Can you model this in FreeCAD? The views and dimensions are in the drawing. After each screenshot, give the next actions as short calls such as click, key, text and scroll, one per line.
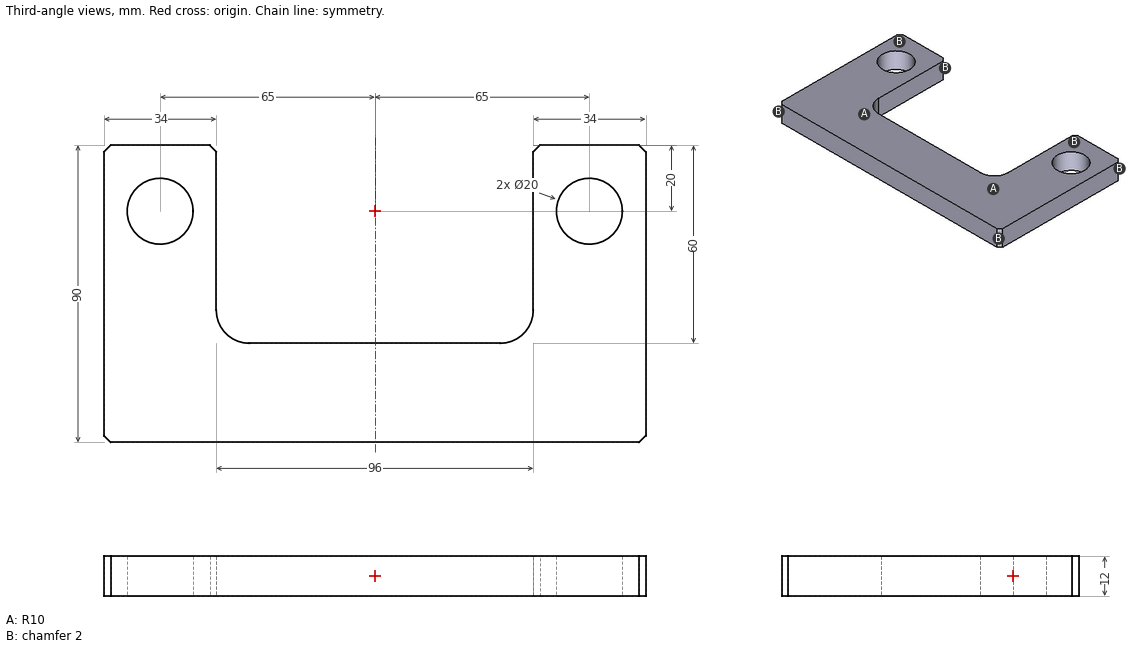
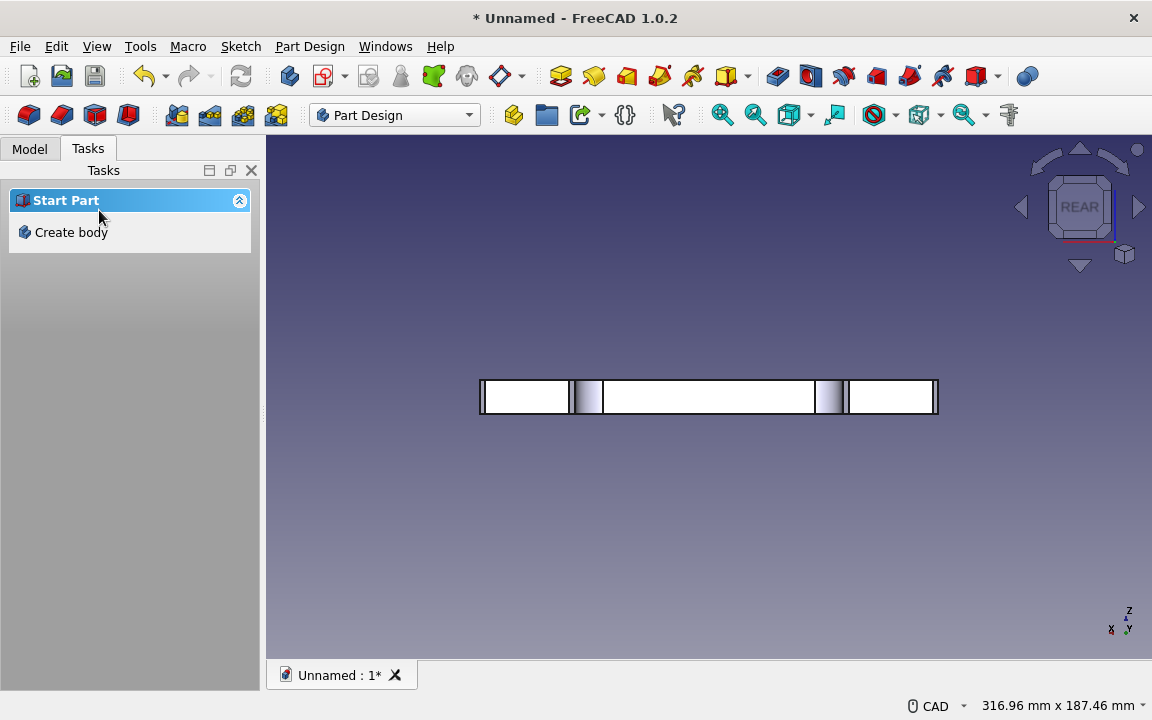
key(0)